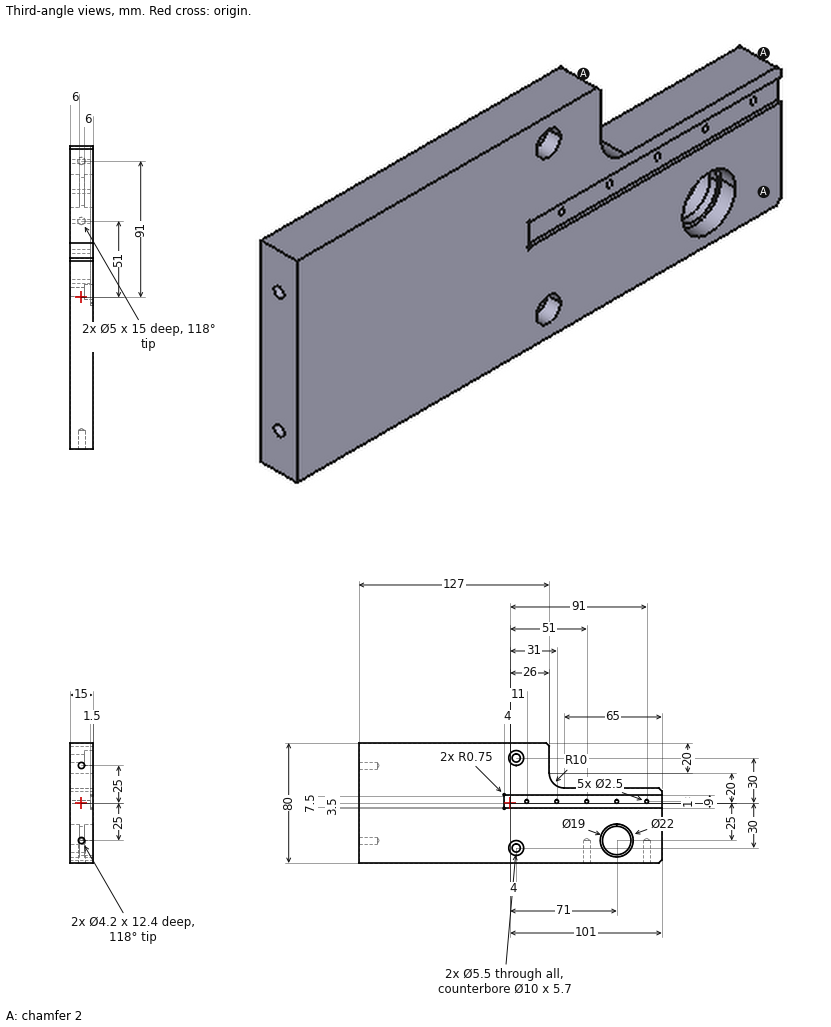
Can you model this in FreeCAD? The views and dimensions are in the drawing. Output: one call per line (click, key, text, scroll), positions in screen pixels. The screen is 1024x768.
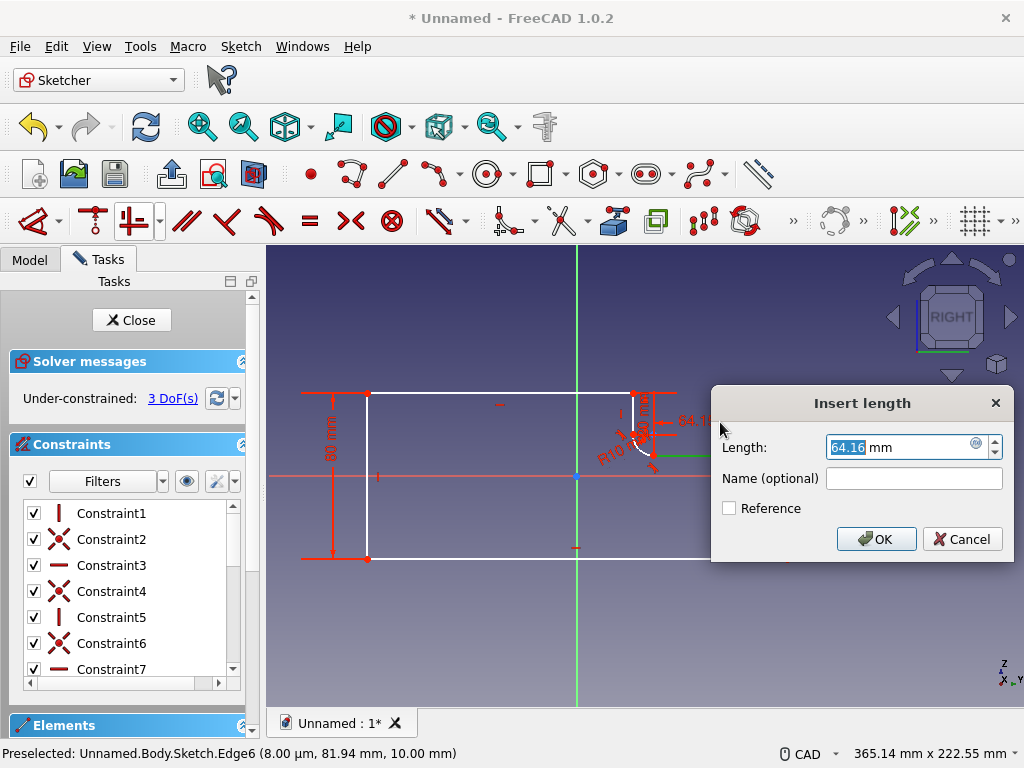
text(65)
key(Return)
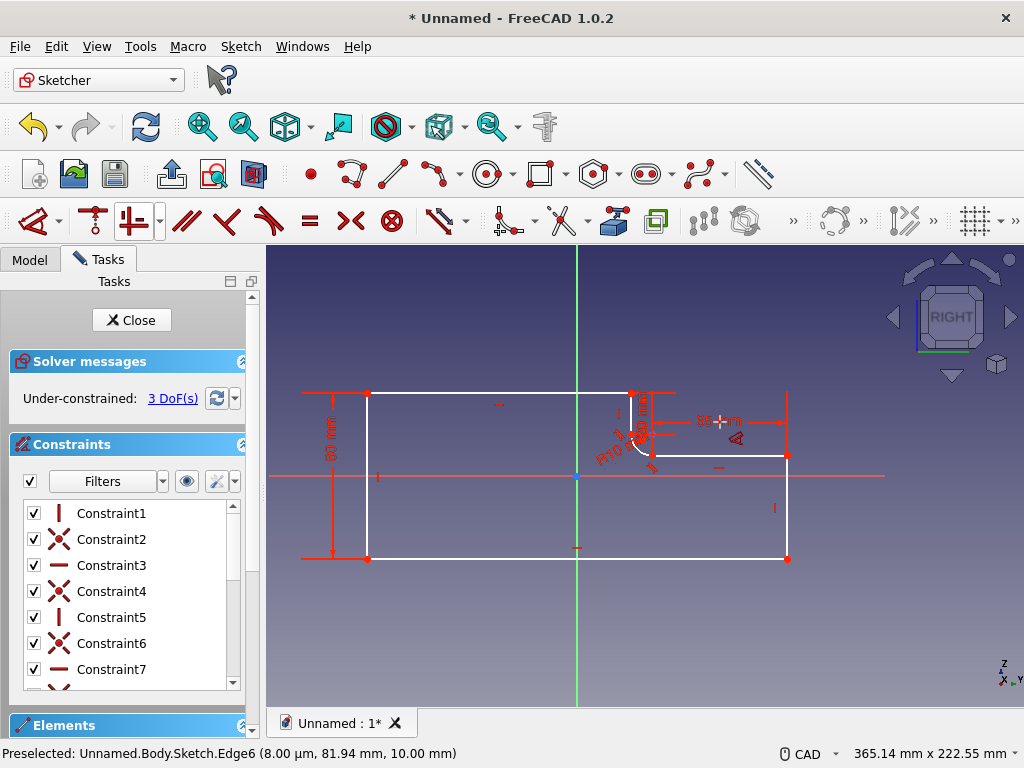
click(552, 393)
click(499, 359)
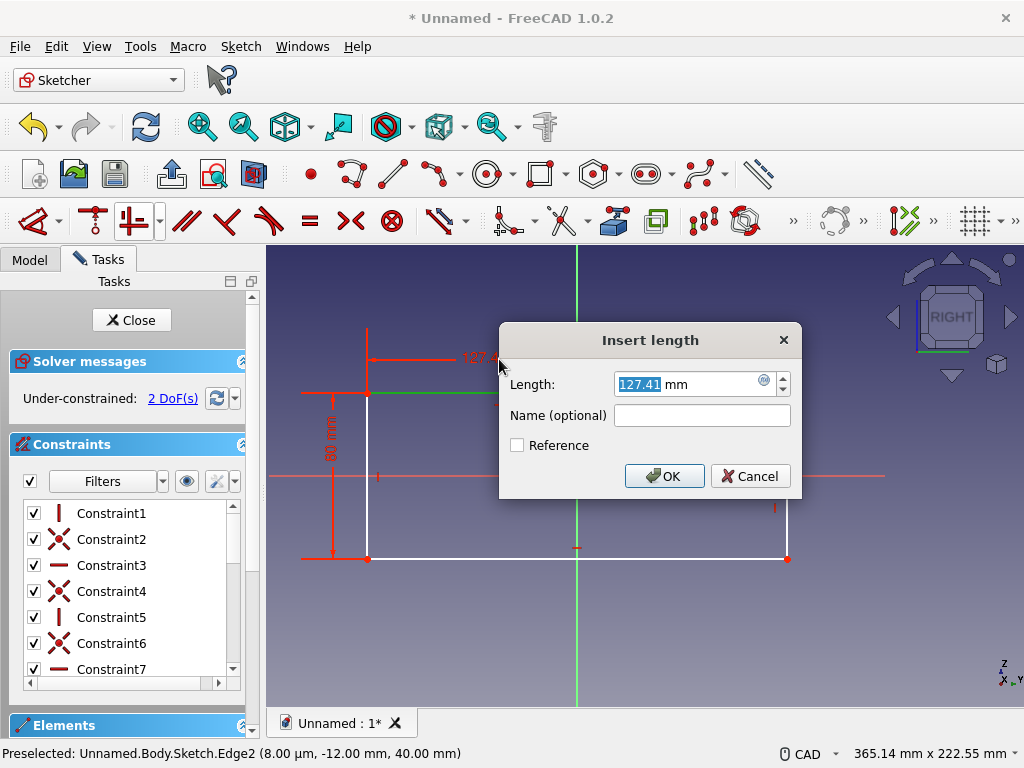
text(127)
key(Return)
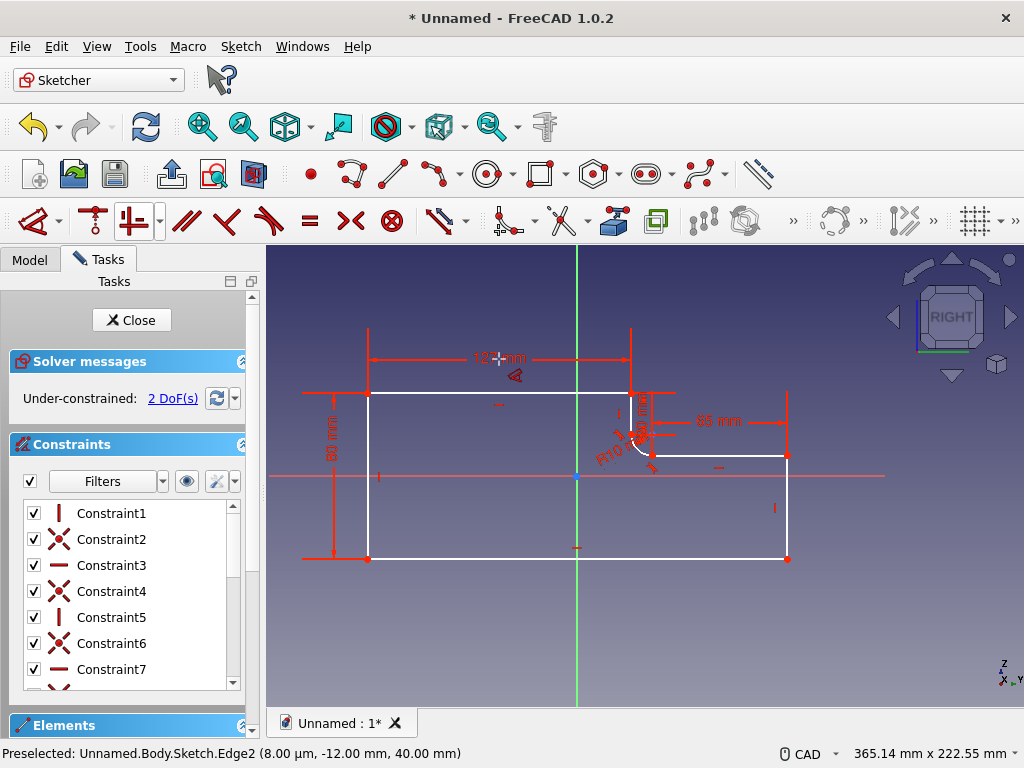
click(631, 435)
click(604, 510)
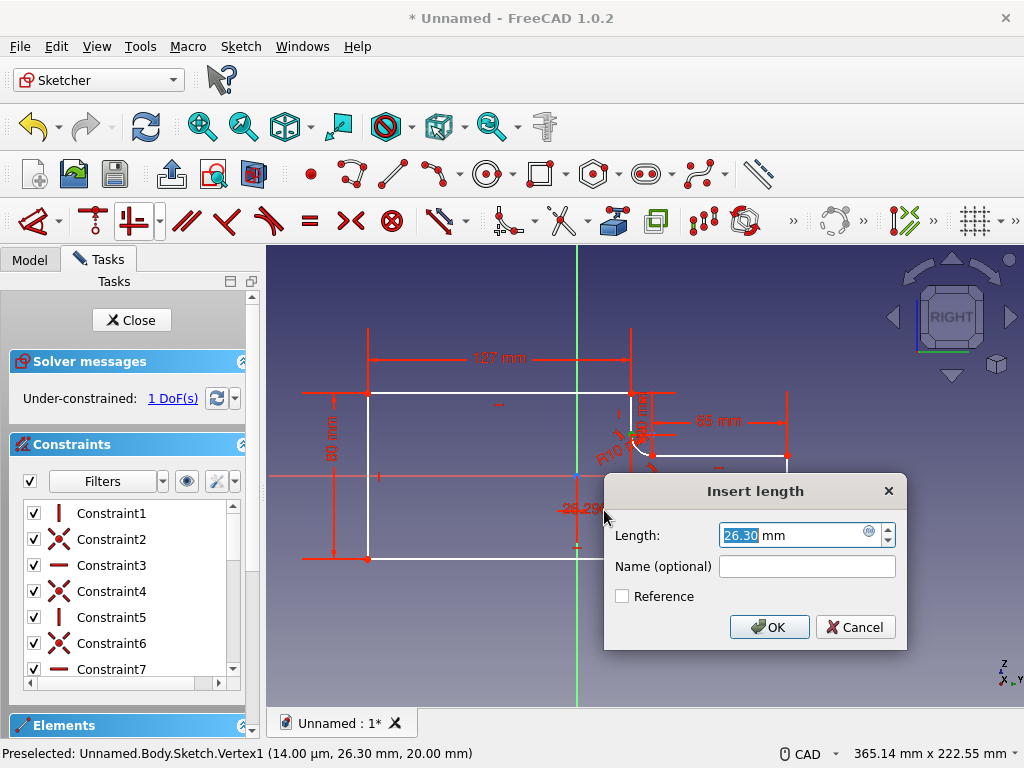
text(26)
key(Return)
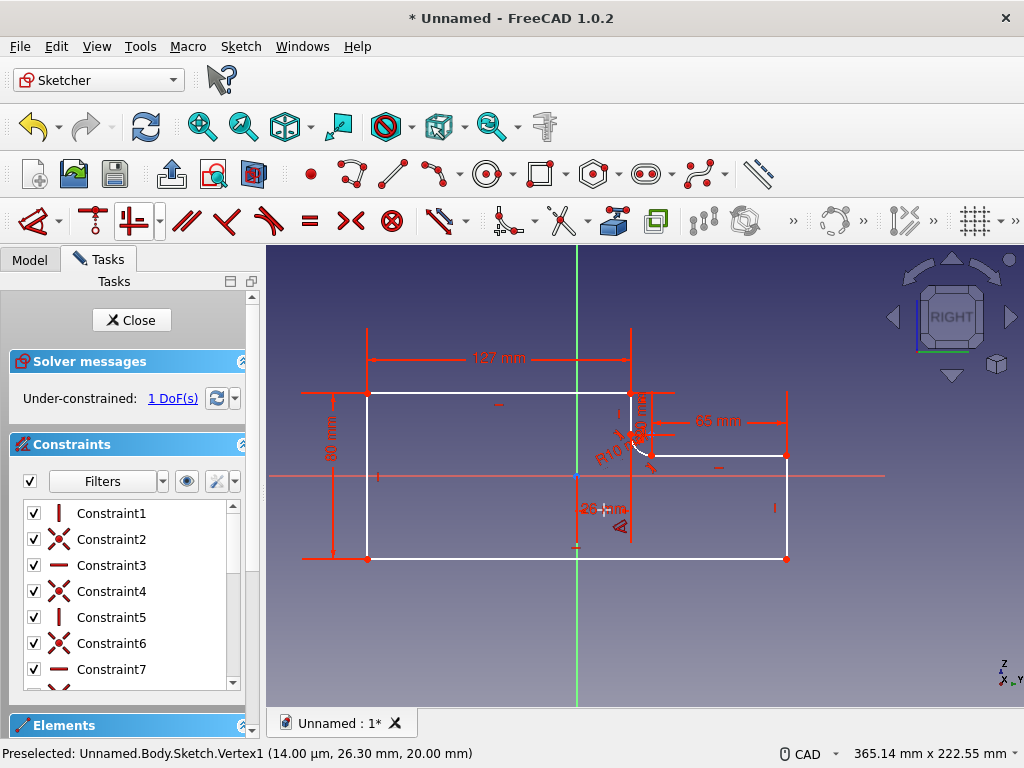
click(631, 435)
click(543, 456)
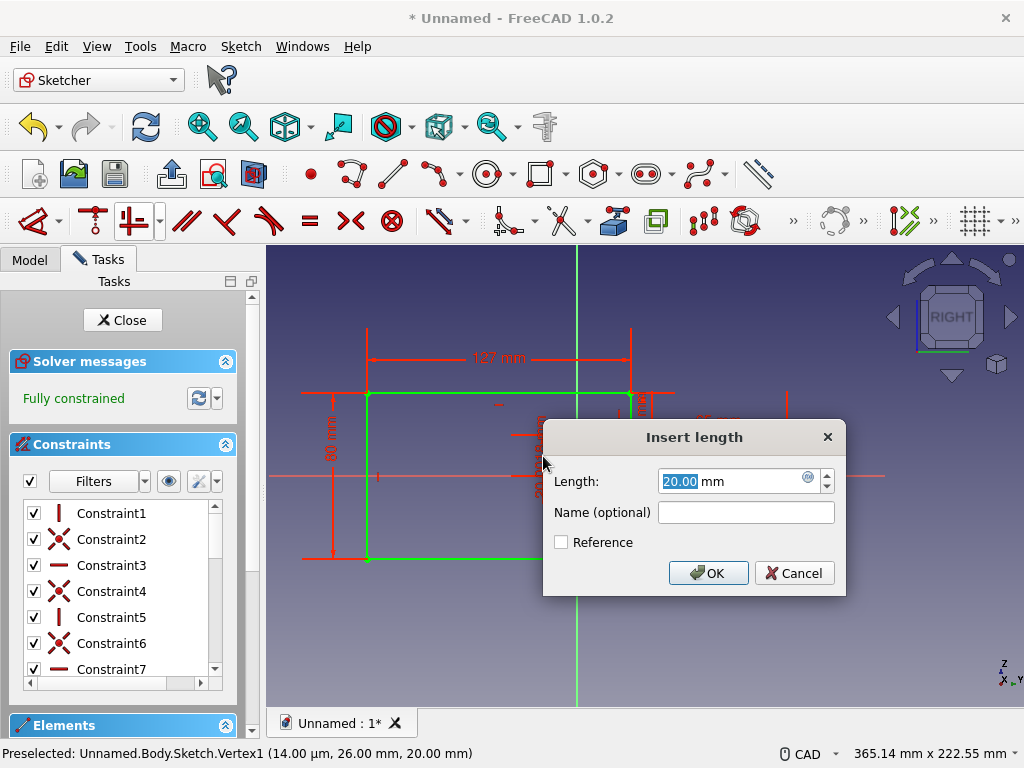
text(20)
key(Return)
key(Escape)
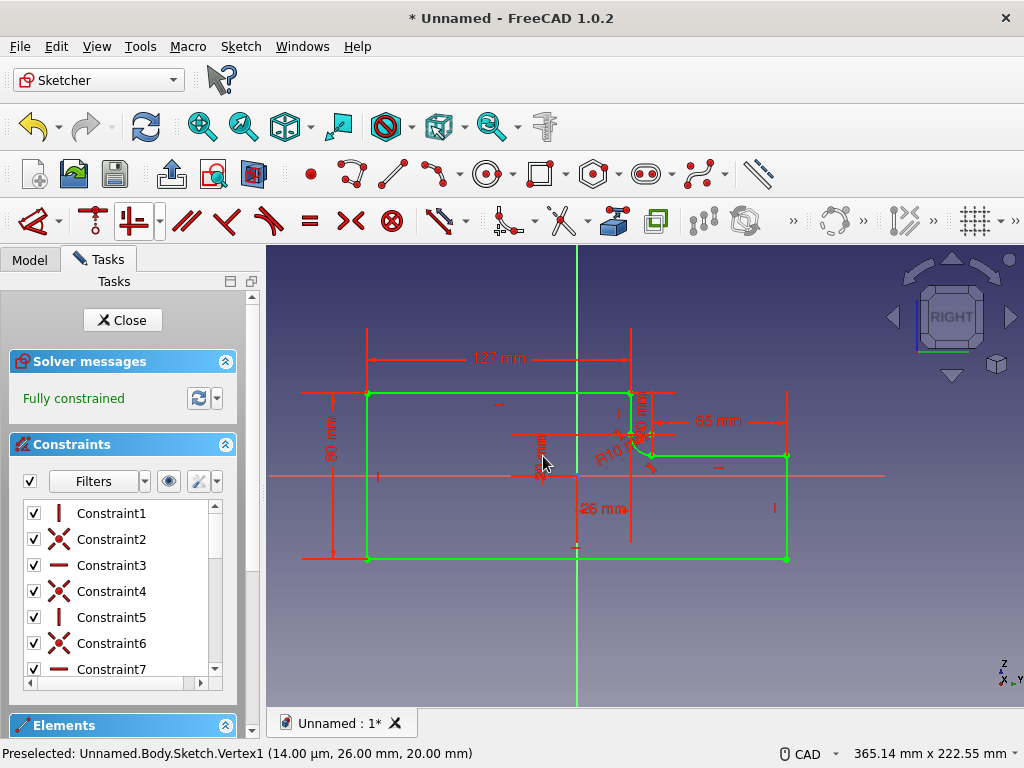
click(123, 320)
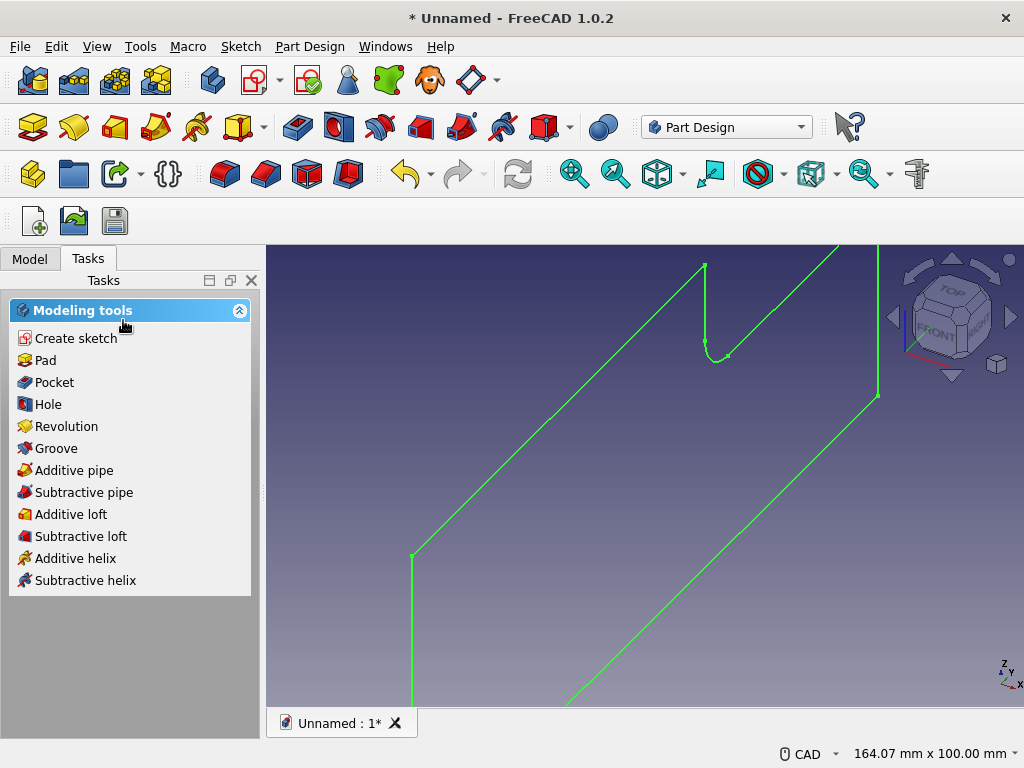
click(33, 128)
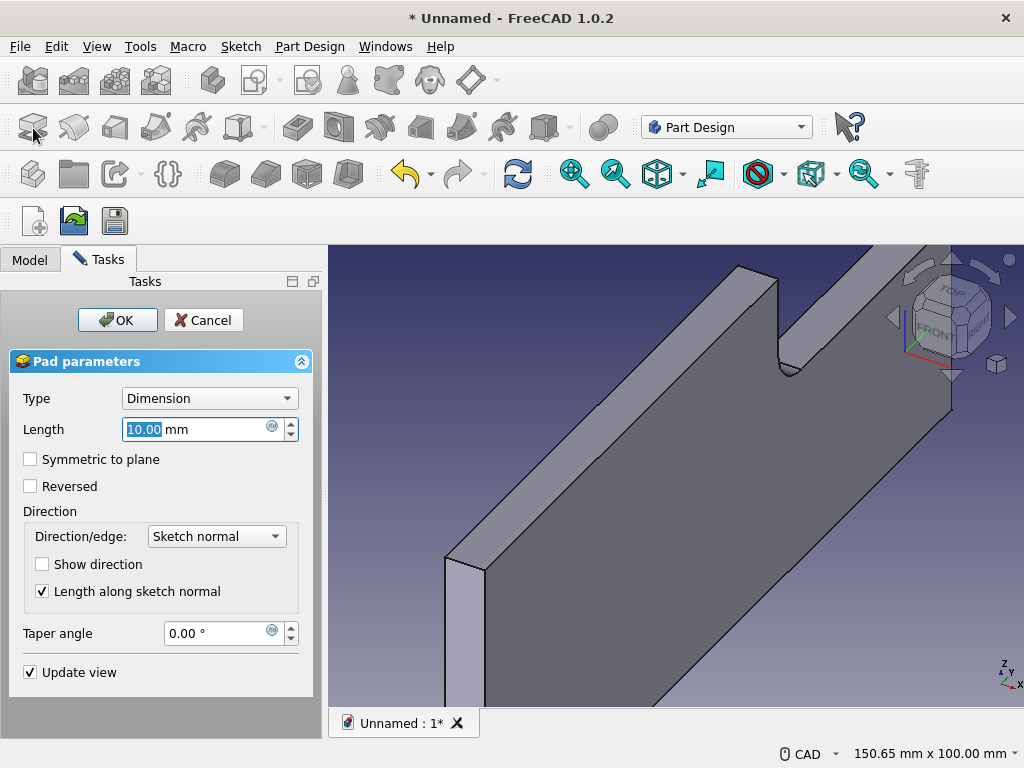
text(15)
key(Tab)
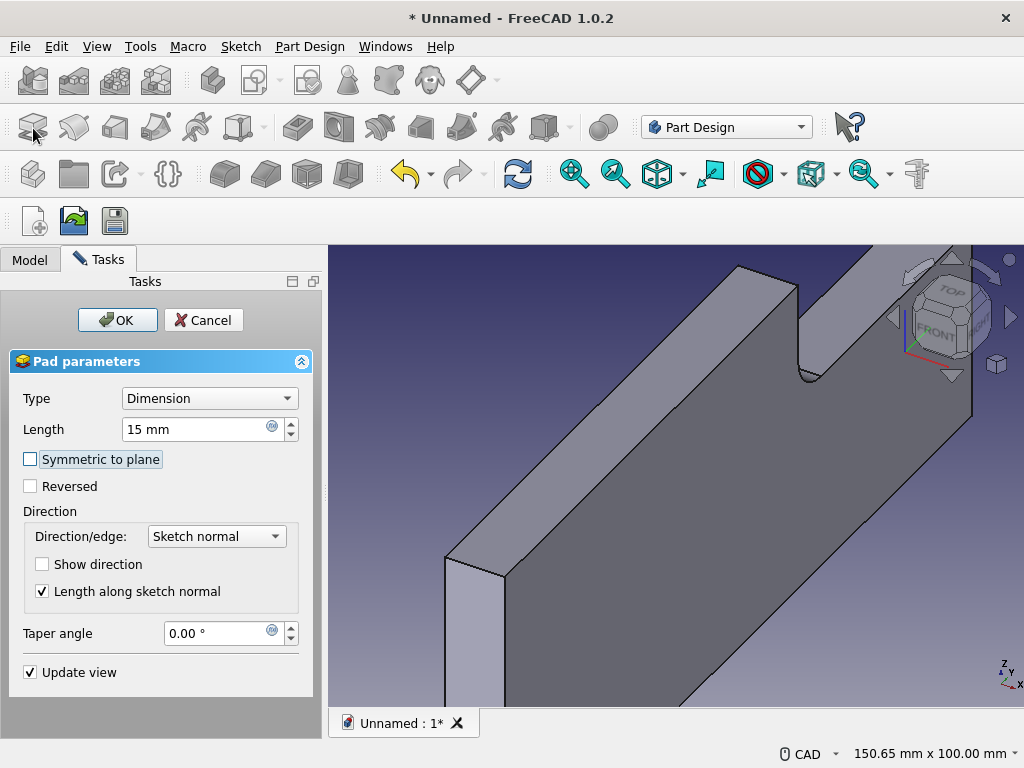
click(31, 459)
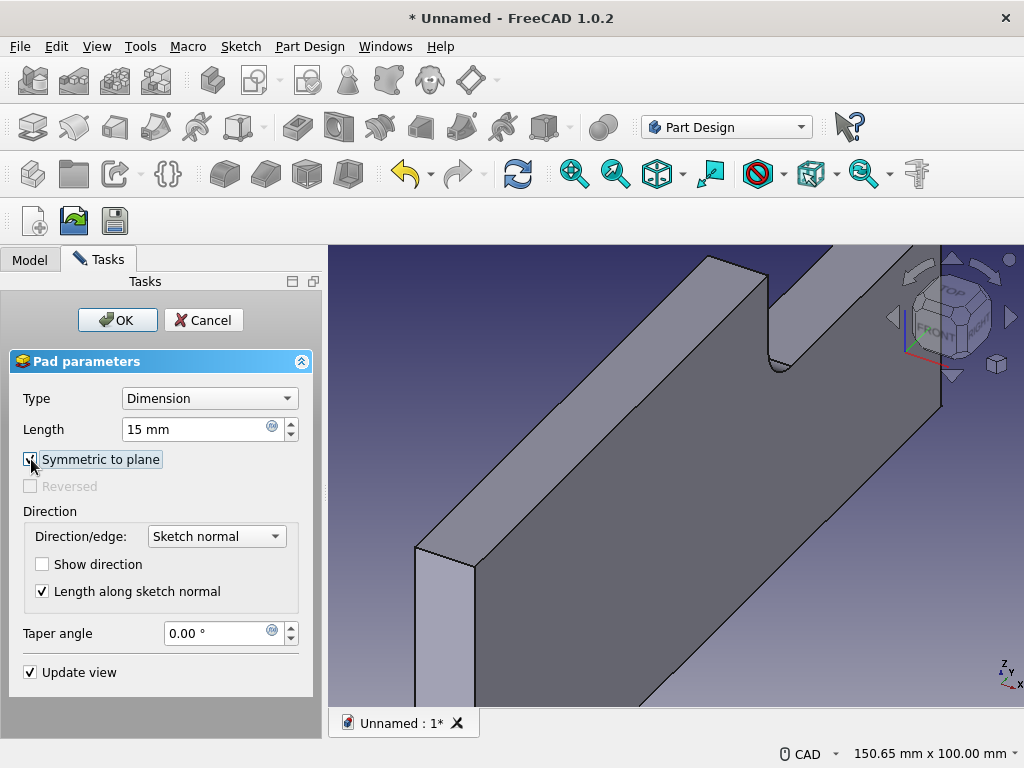
click(118, 320)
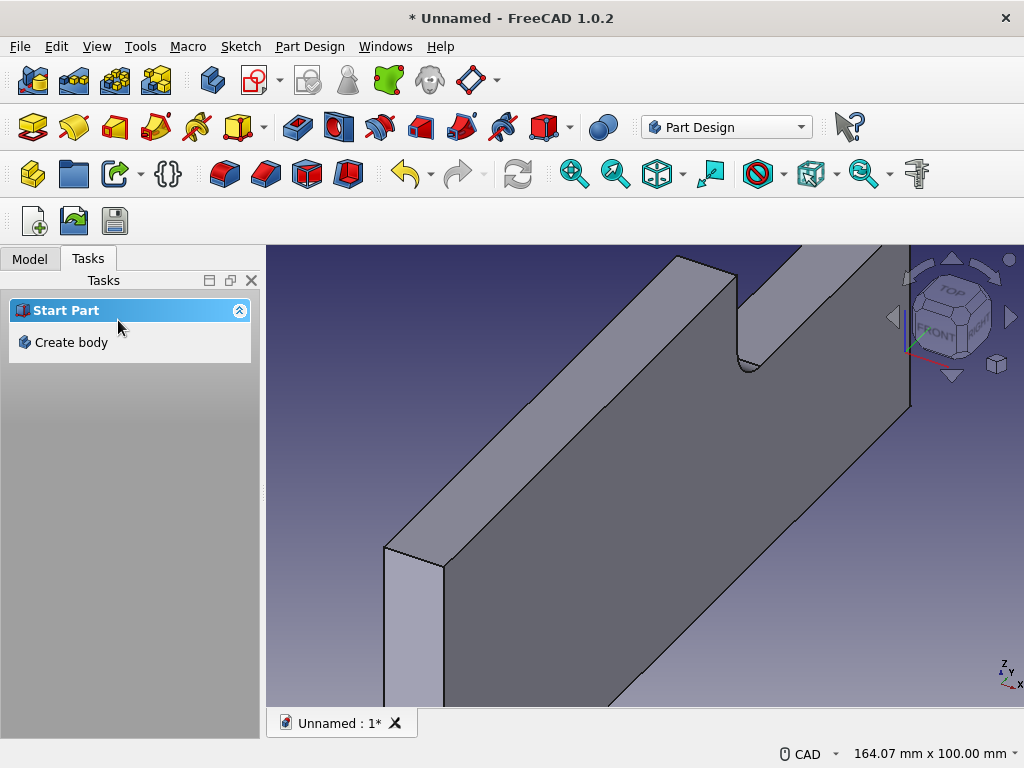
key(v)
key(f)